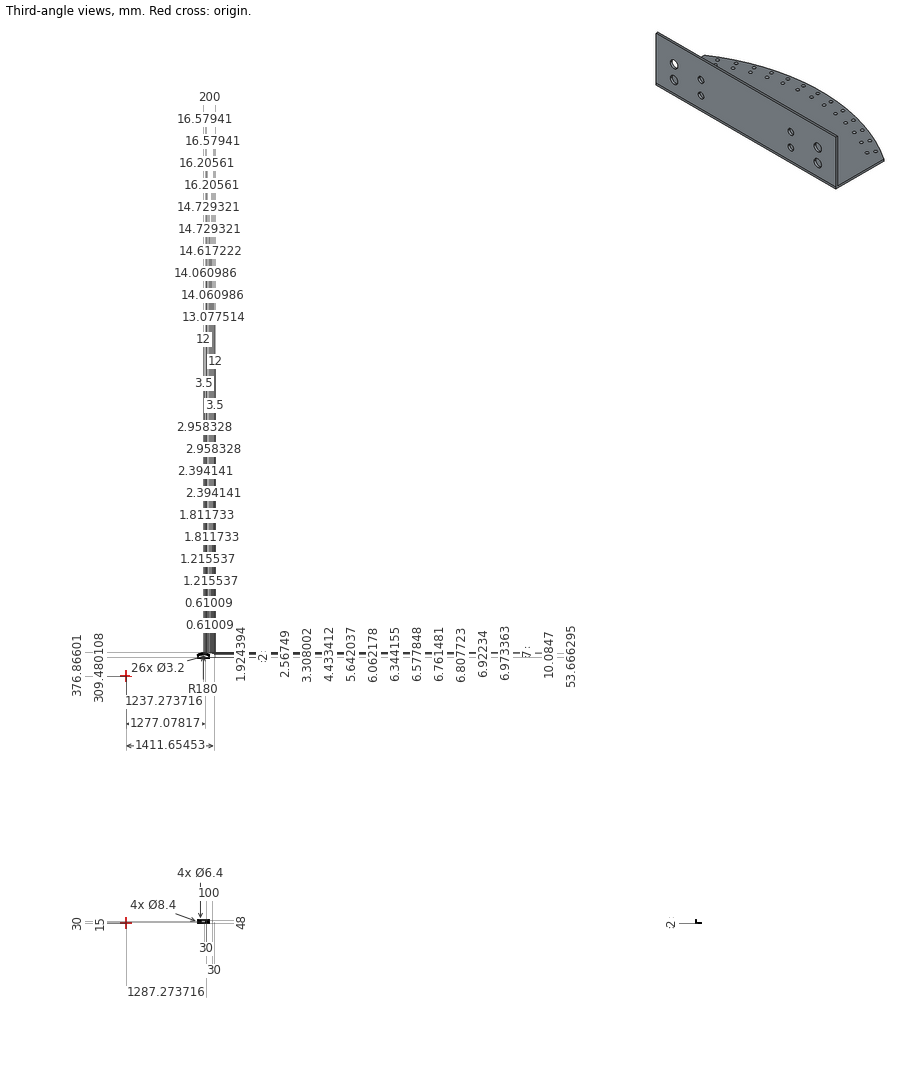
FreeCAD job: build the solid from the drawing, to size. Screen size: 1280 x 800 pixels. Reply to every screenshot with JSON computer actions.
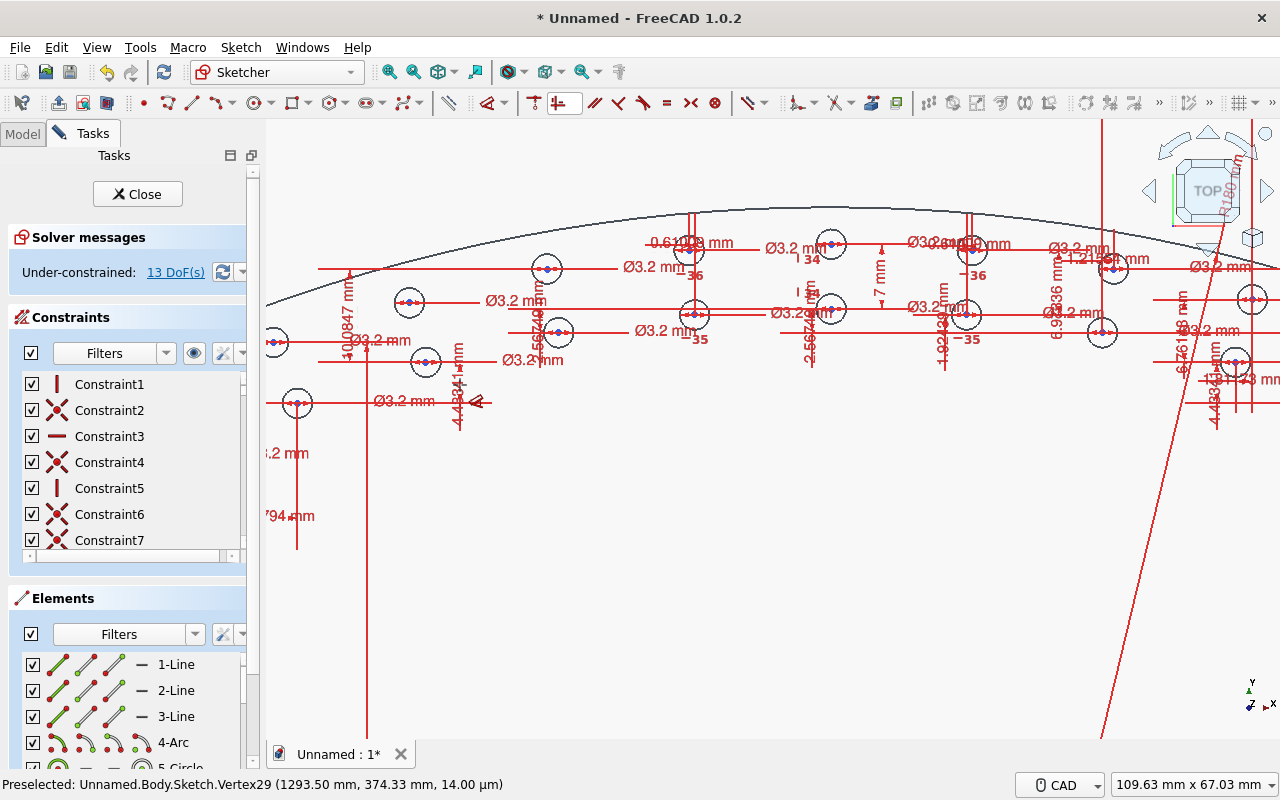
{"action": "scroll", "coordinate": [297, 403], "scroll_direction": "up", "scroll_amount": 3}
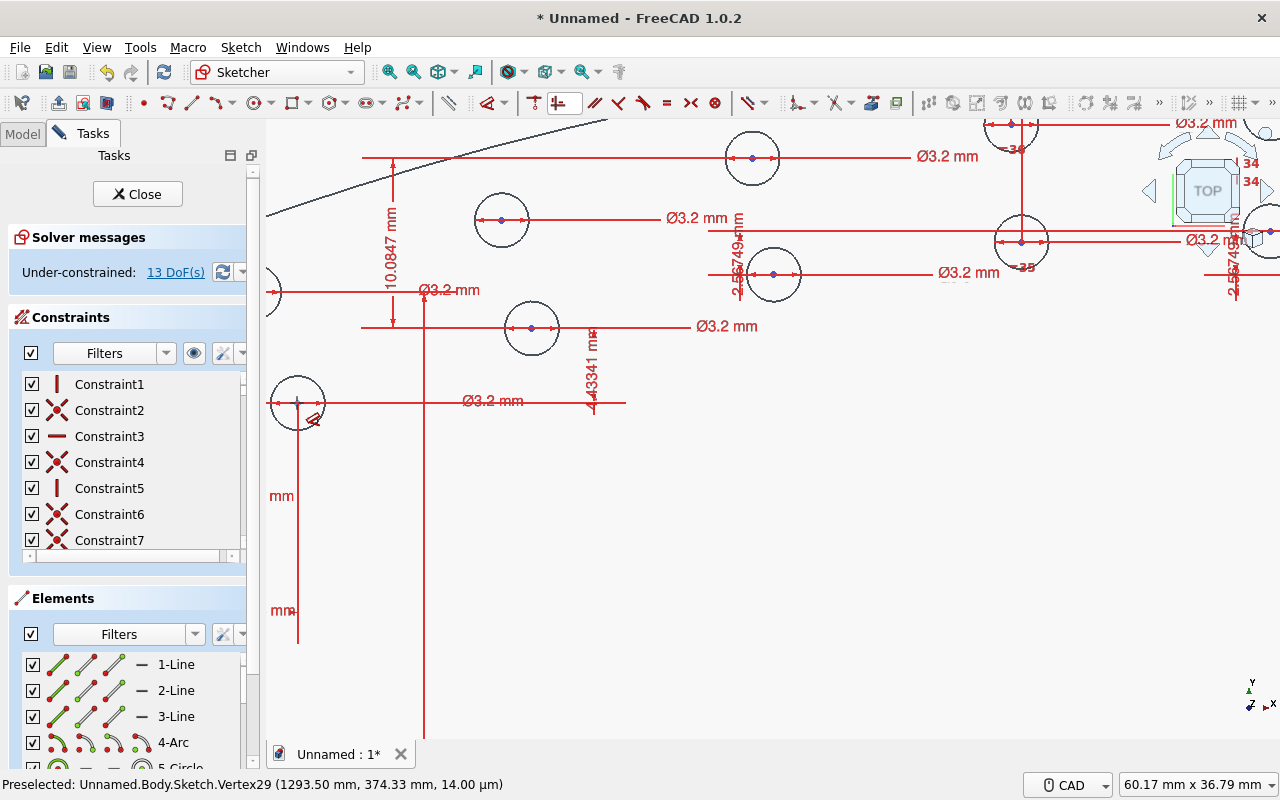
{"action": "left_click", "coordinate": [298, 403]}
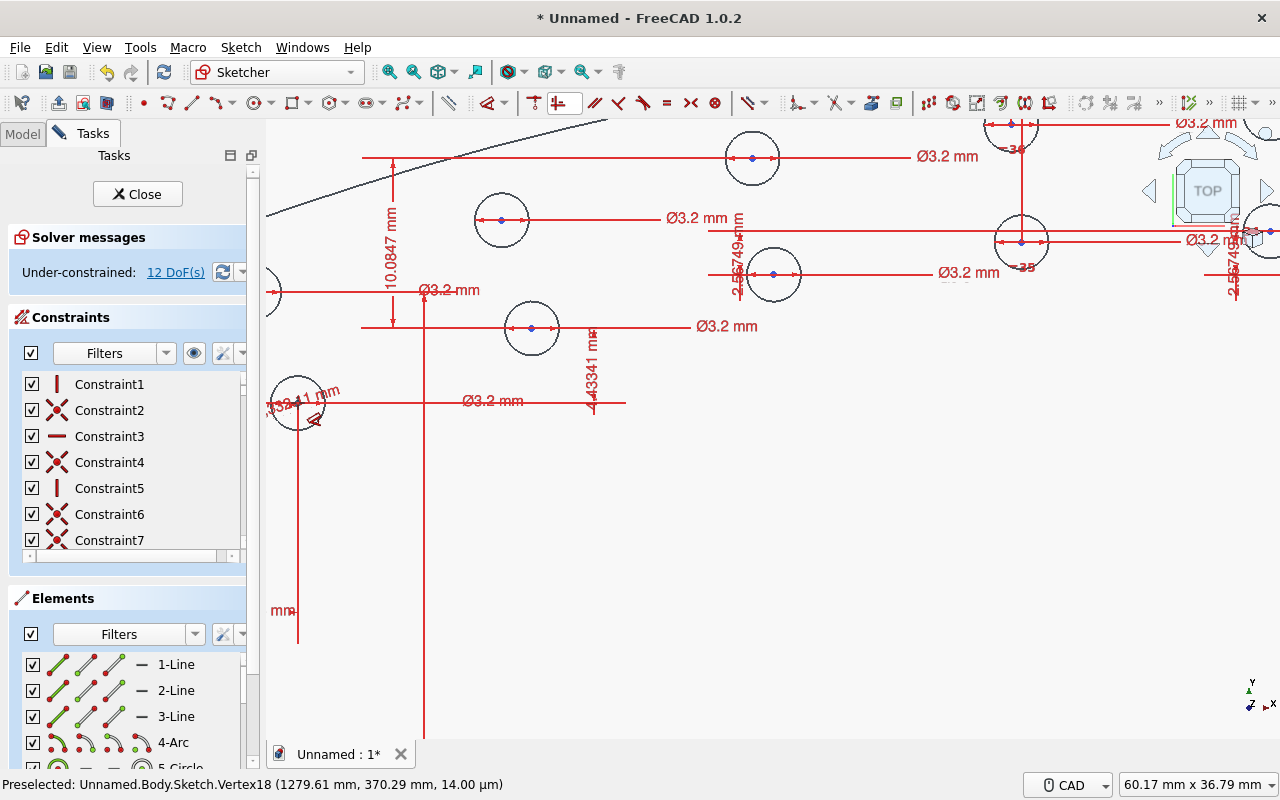
{"action": "scroll", "coordinate": [593, 365], "scroll_direction": "down", "scroll_amount": 9}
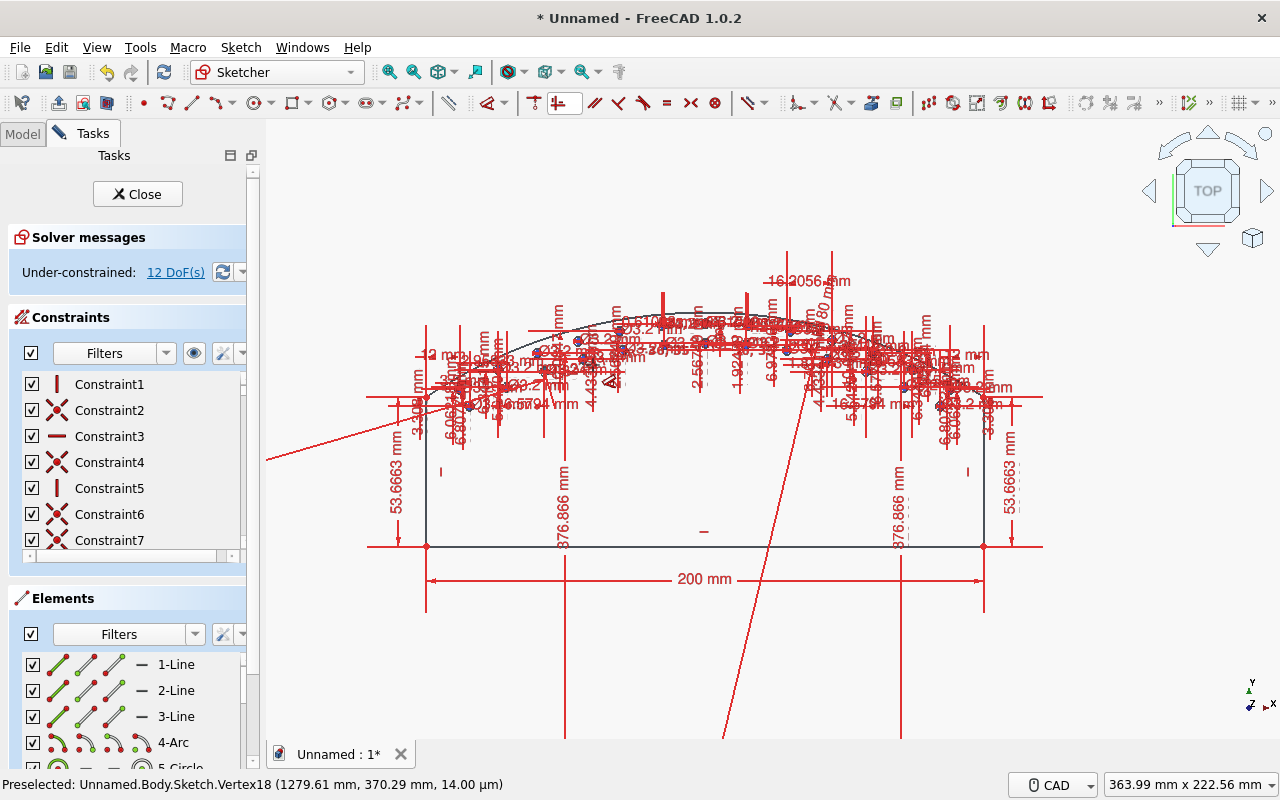
{"action": "scroll", "coordinate": [537, 353], "scroll_direction": "up", "scroll_amount": 9}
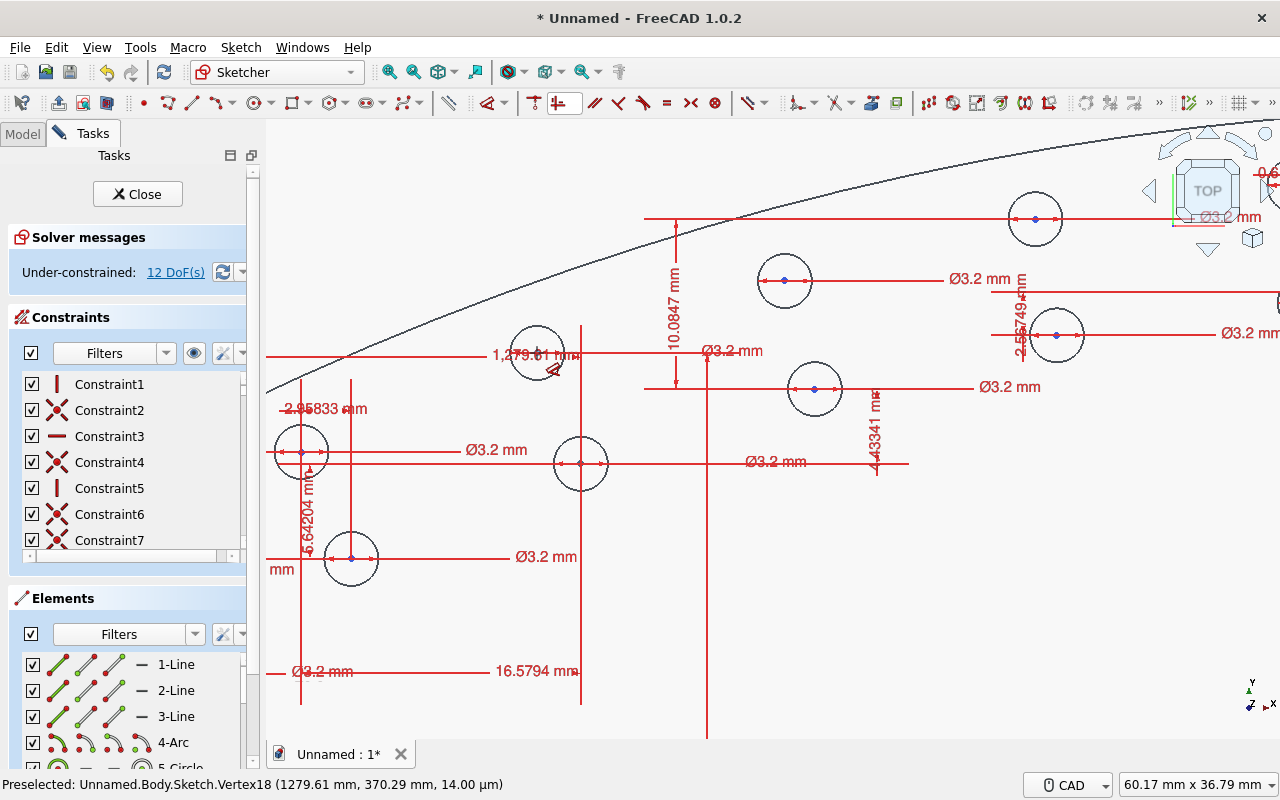
{"action": "left_click", "coordinate": [537, 353]}
{"action": "left_click", "coordinate": [559, 319]}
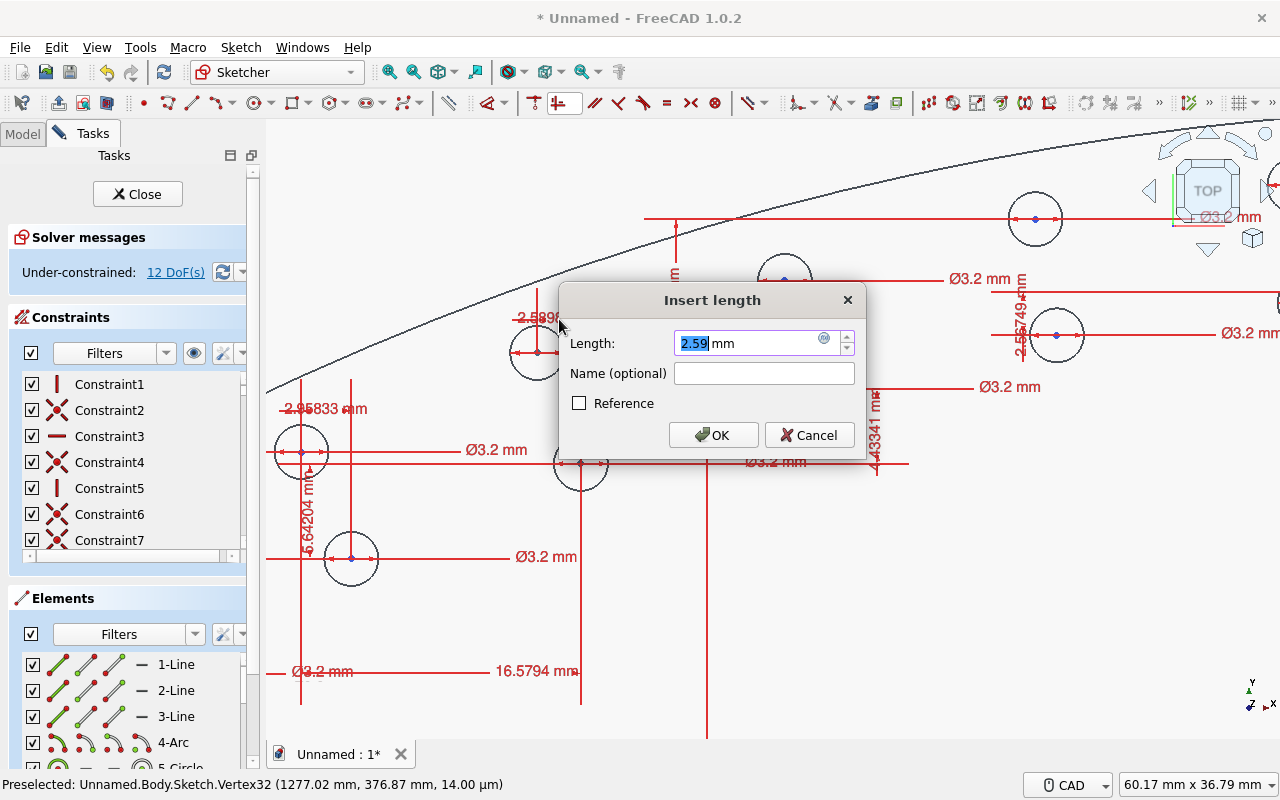
{"action": "type", "text": "2.394141"}
{"action": "key", "text": "Return"}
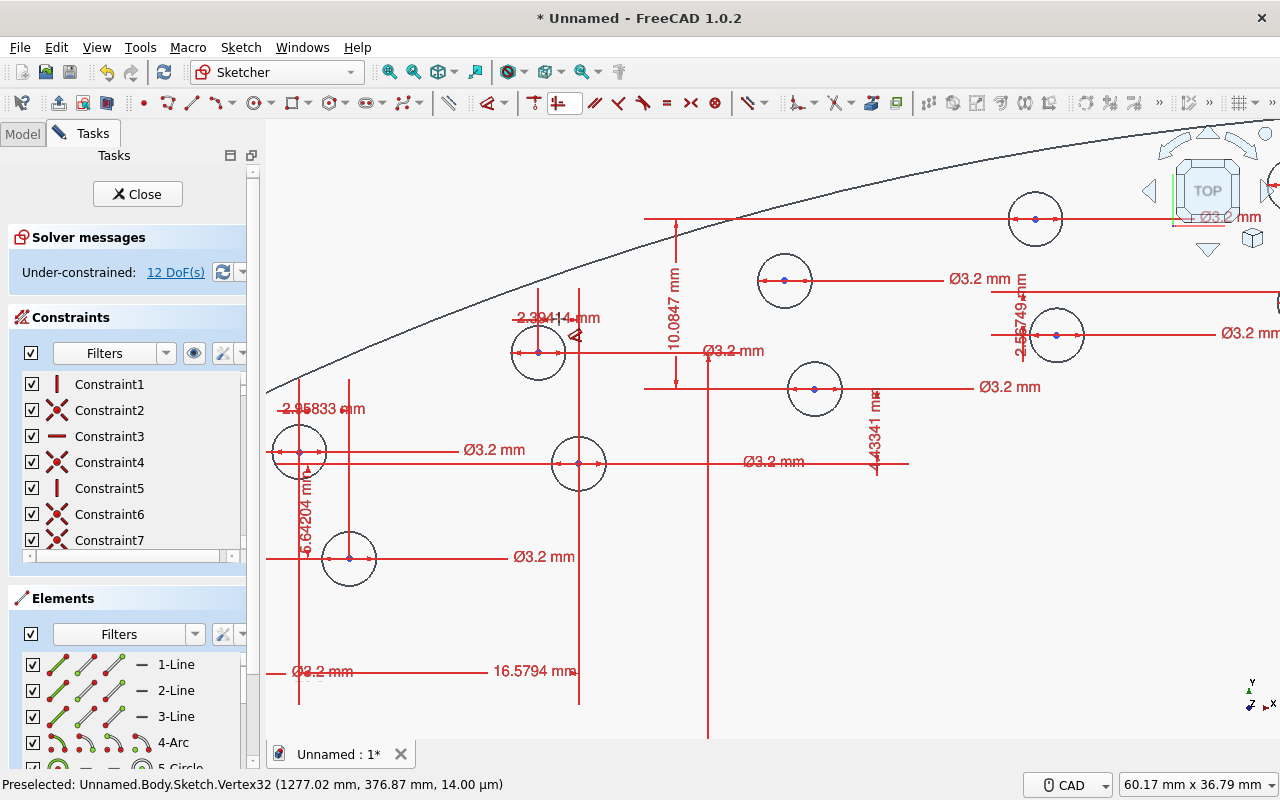
{"action": "scroll", "coordinate": [1057, 335], "scroll_direction": "up", "scroll_amount": 4}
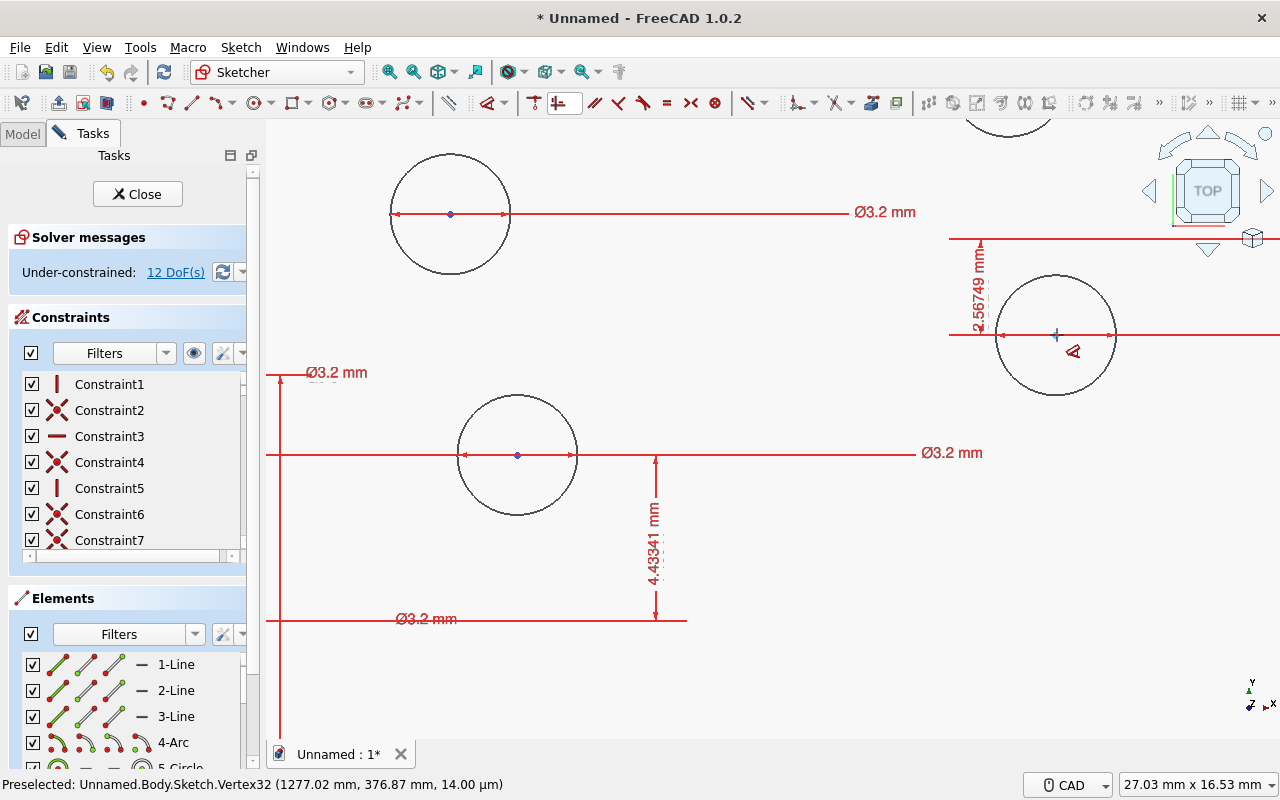
{"action": "left_click", "coordinate": [1056, 335]}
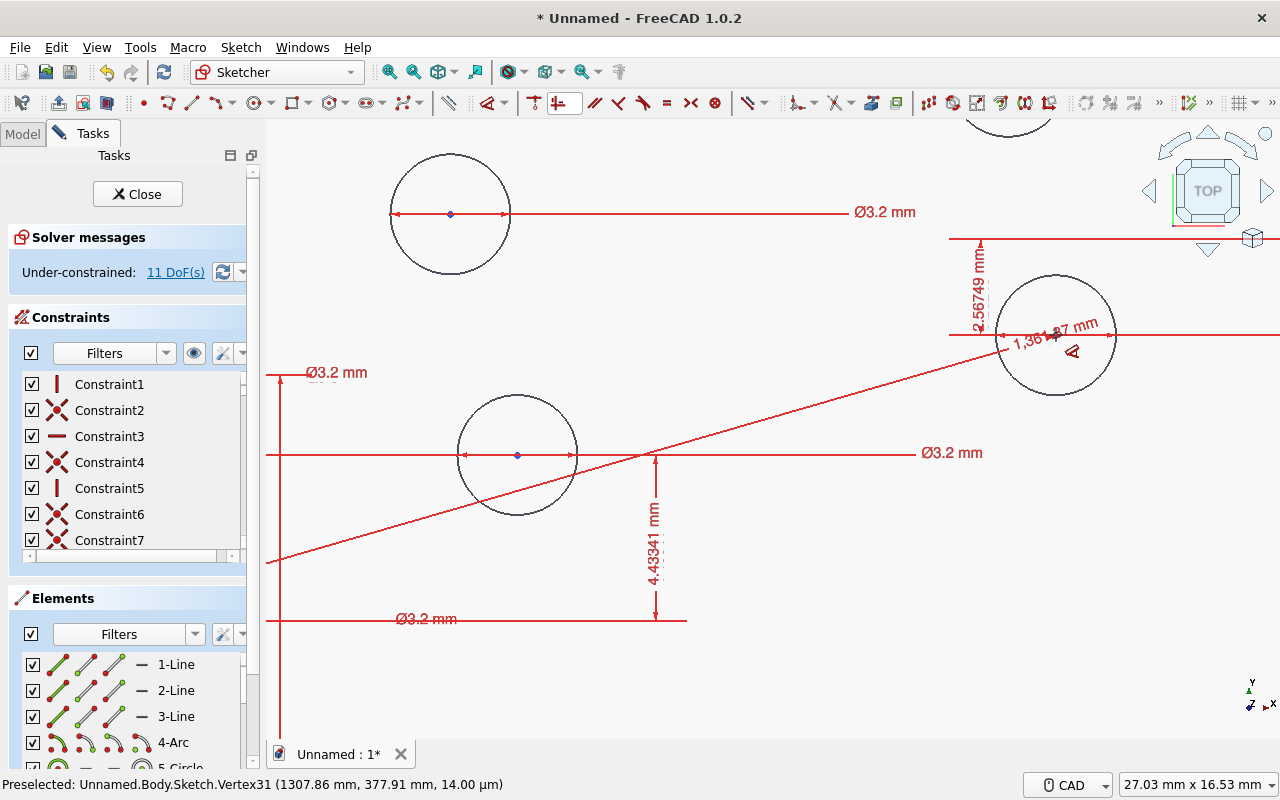
{"action": "scroll", "coordinate": [588, 351], "scroll_direction": "down", "scroll_amount": 13}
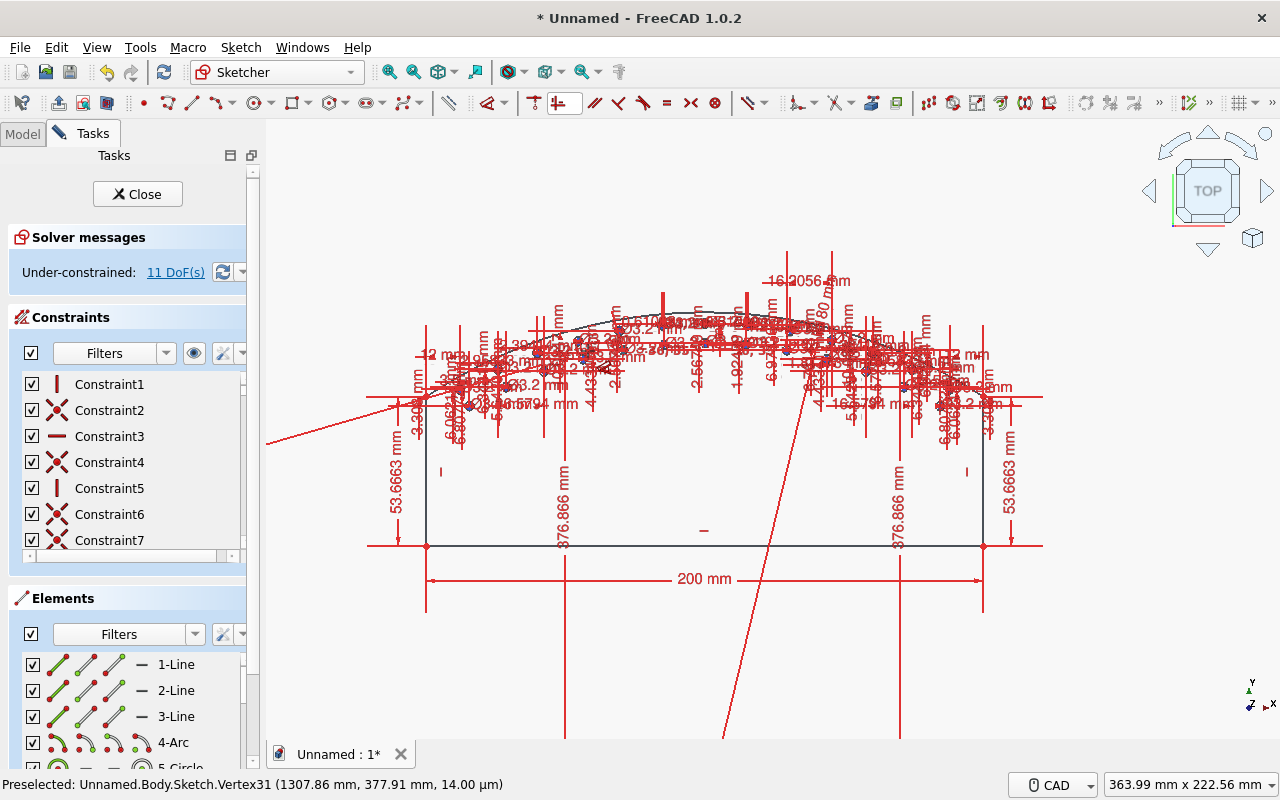
{"action": "scroll", "coordinate": [620, 331], "scroll_direction": "up", "scroll_amount": 13}